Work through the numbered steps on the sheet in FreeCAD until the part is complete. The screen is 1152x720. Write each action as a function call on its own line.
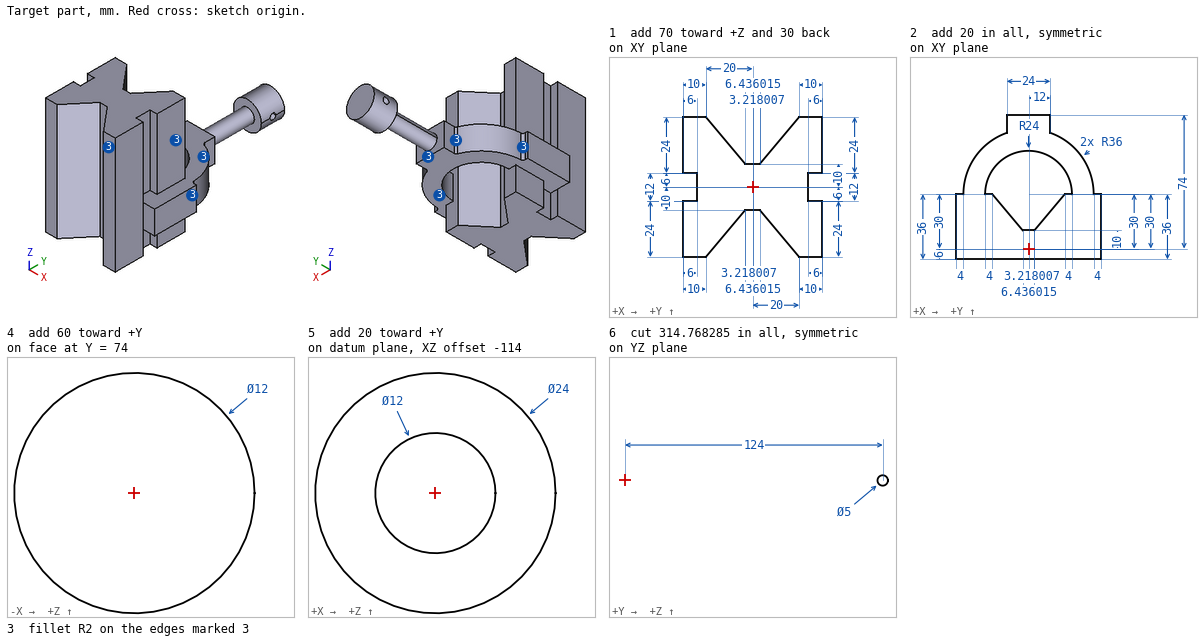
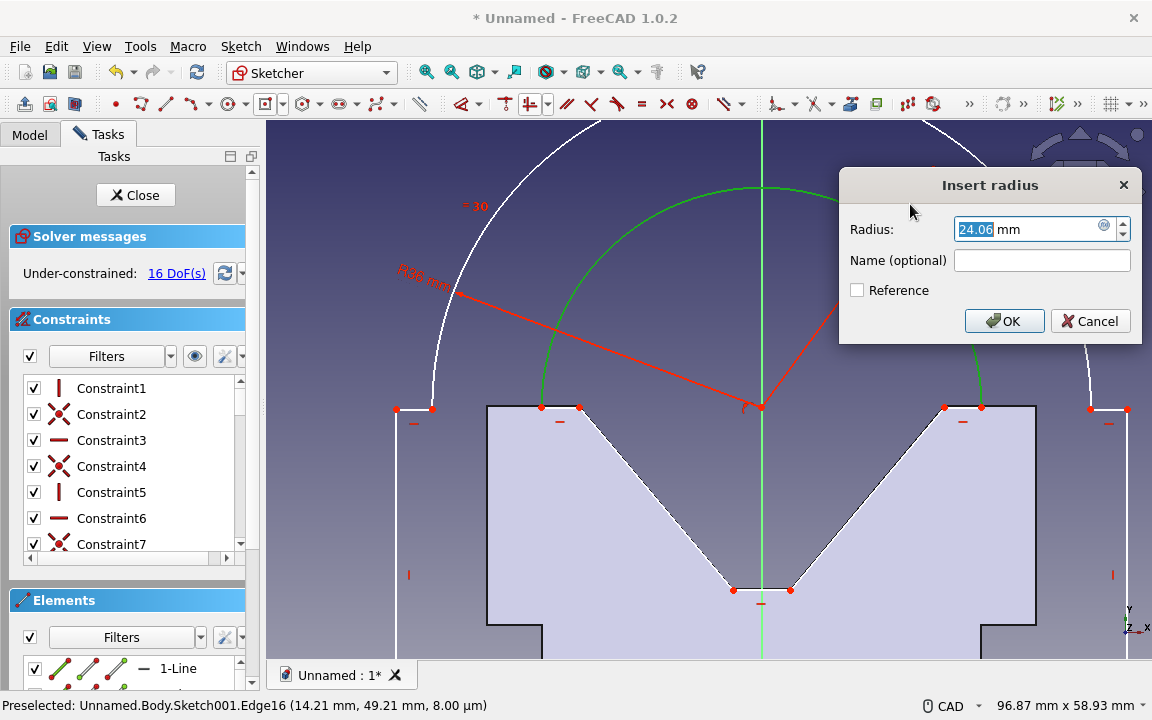
text(24)
key(Return)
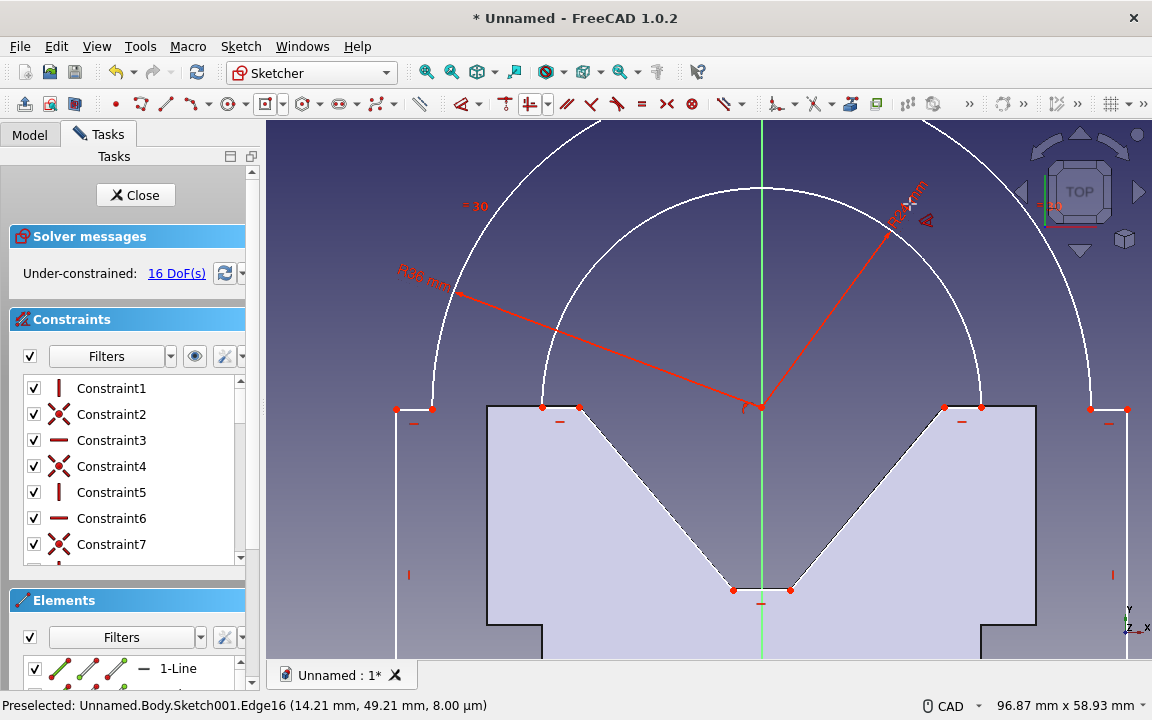
scroll(421, 410, up, 2)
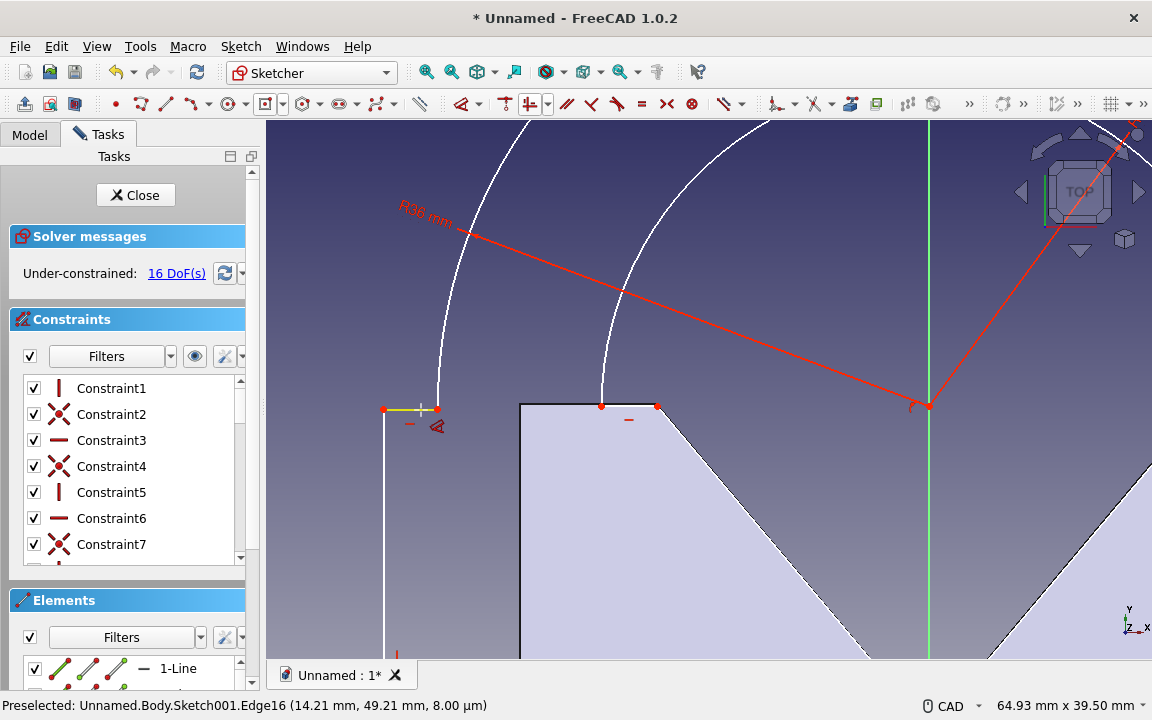
click(422, 410)
click(411, 444)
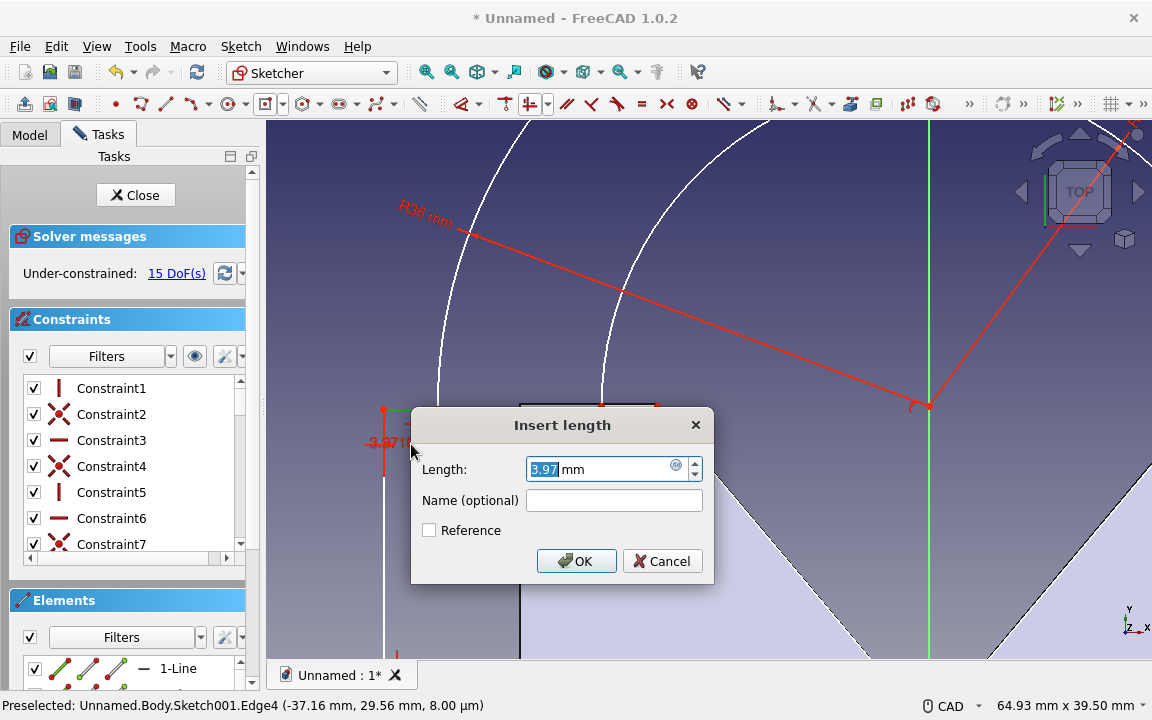
text(4)
key(Return)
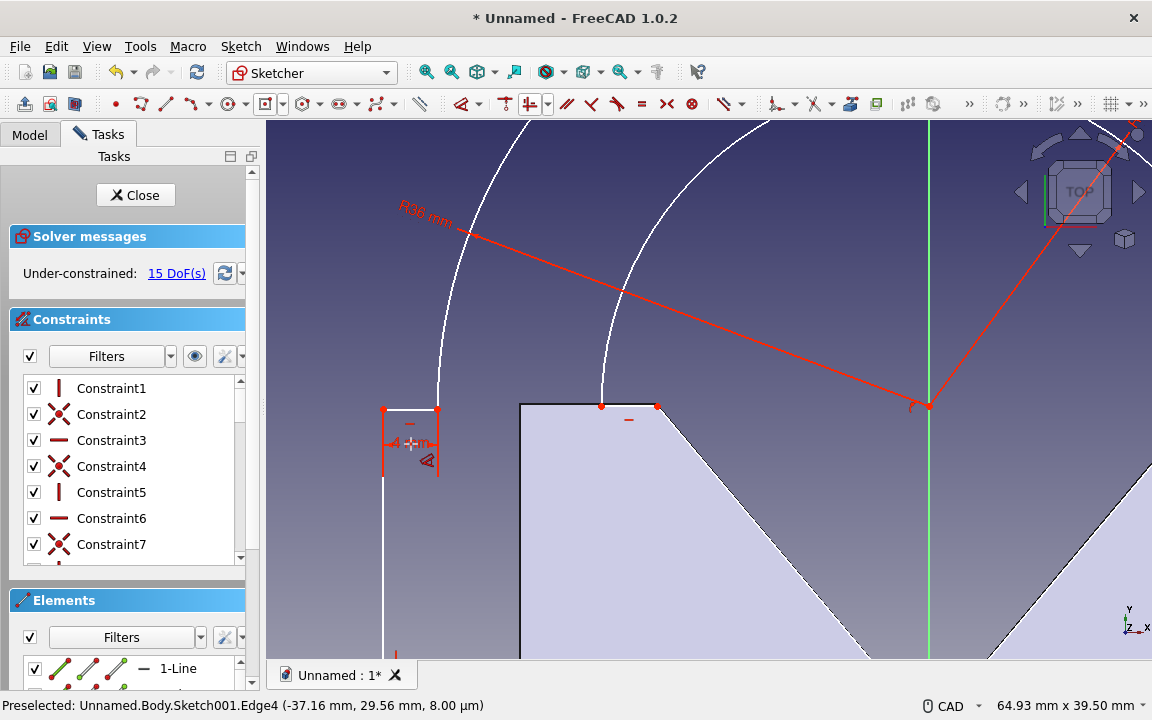
scroll(516, 407, down, 6)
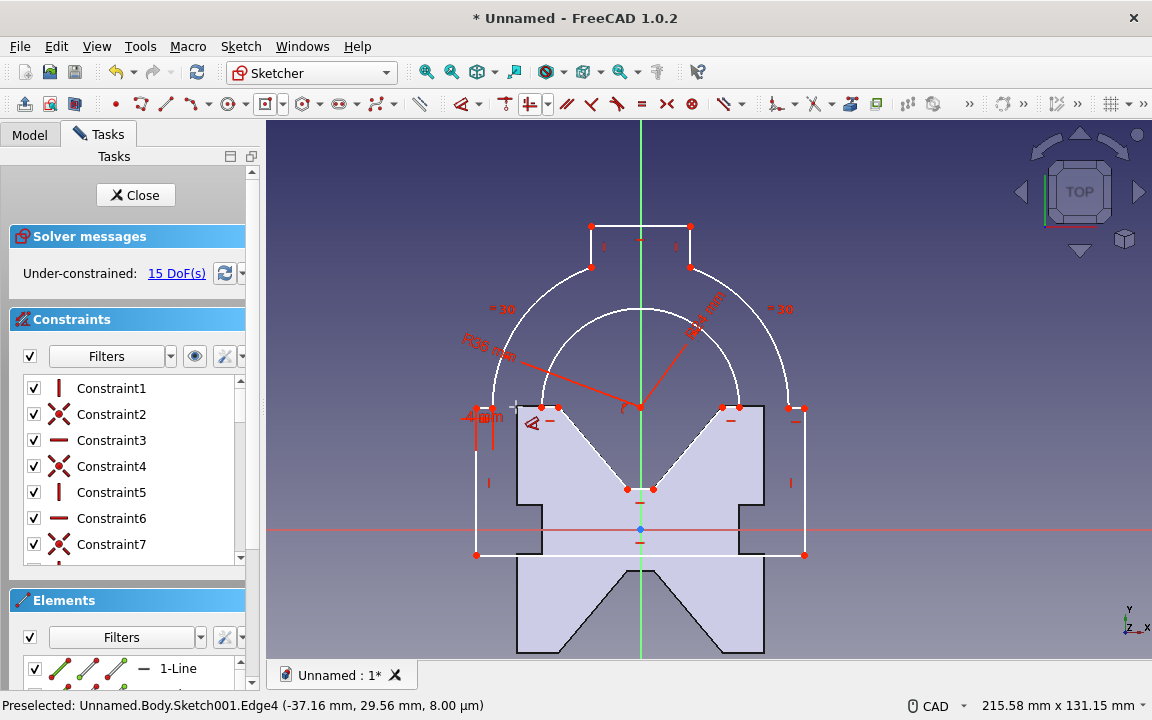
scroll(800, 408, up, 6)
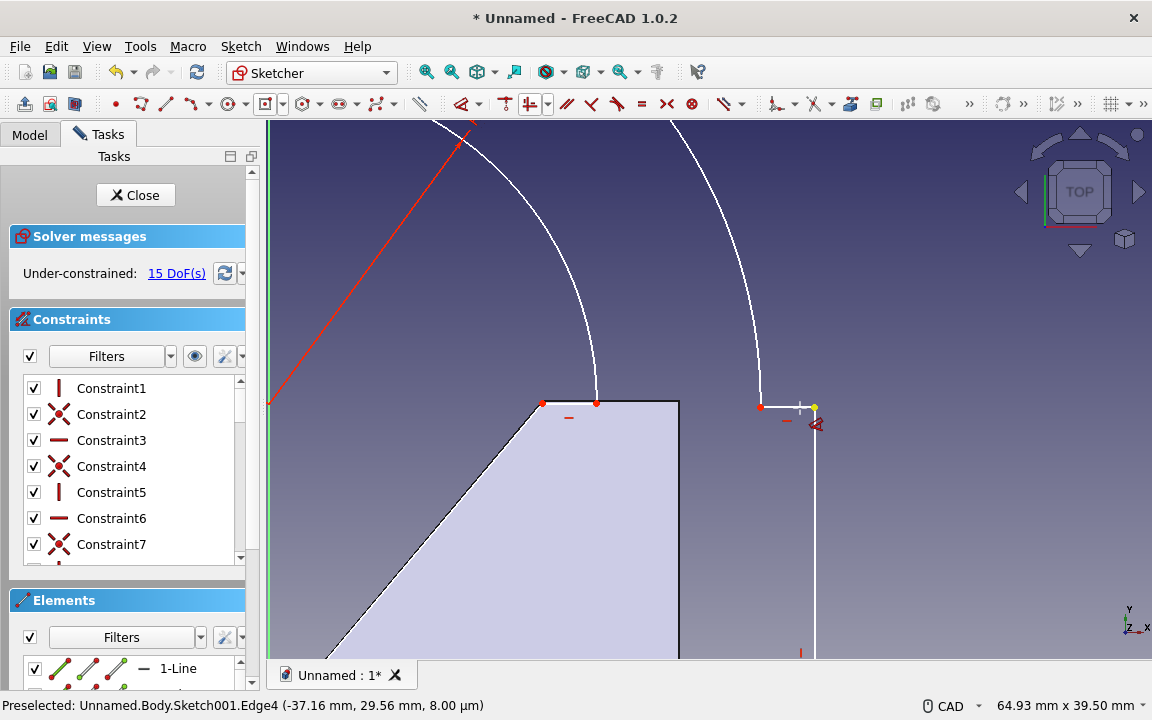
click(799, 407)
click(788, 441)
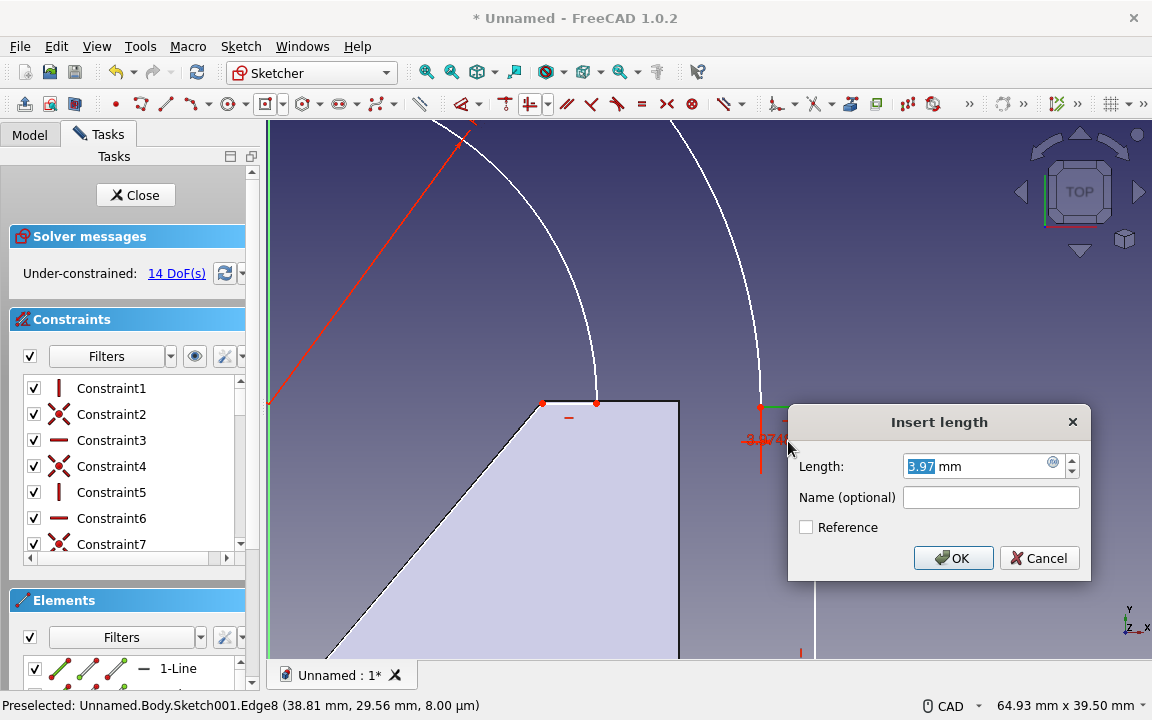
text(4)
key(Return)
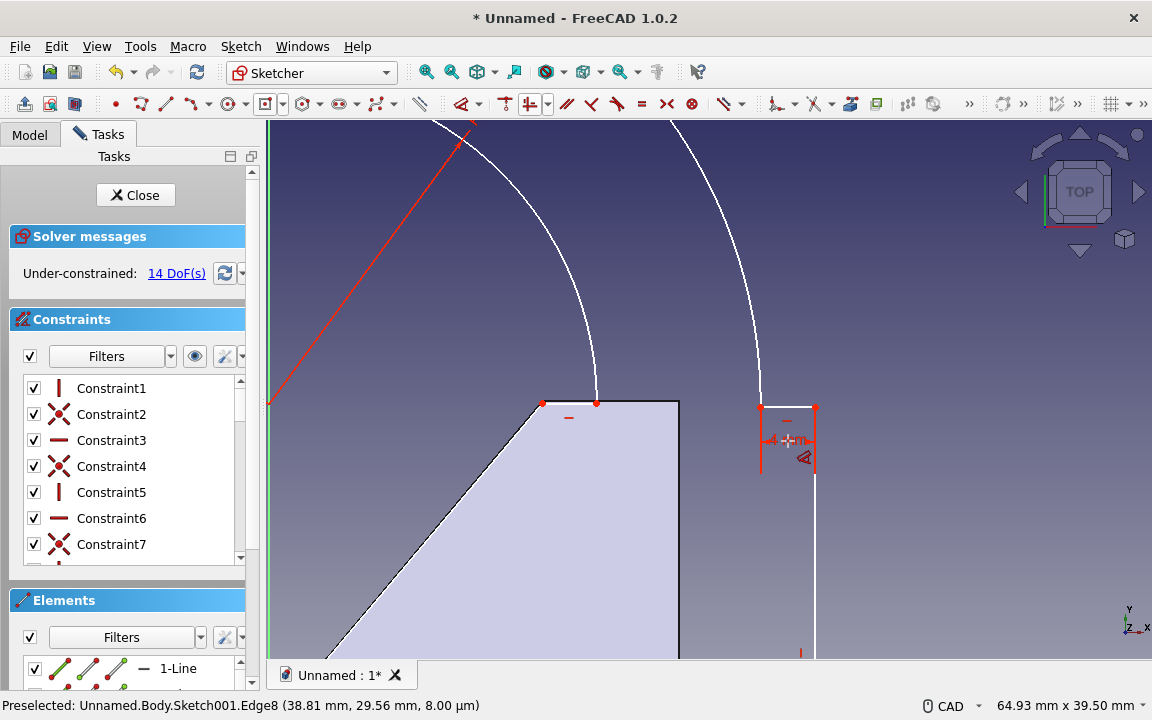
click(580, 404)
click(570, 438)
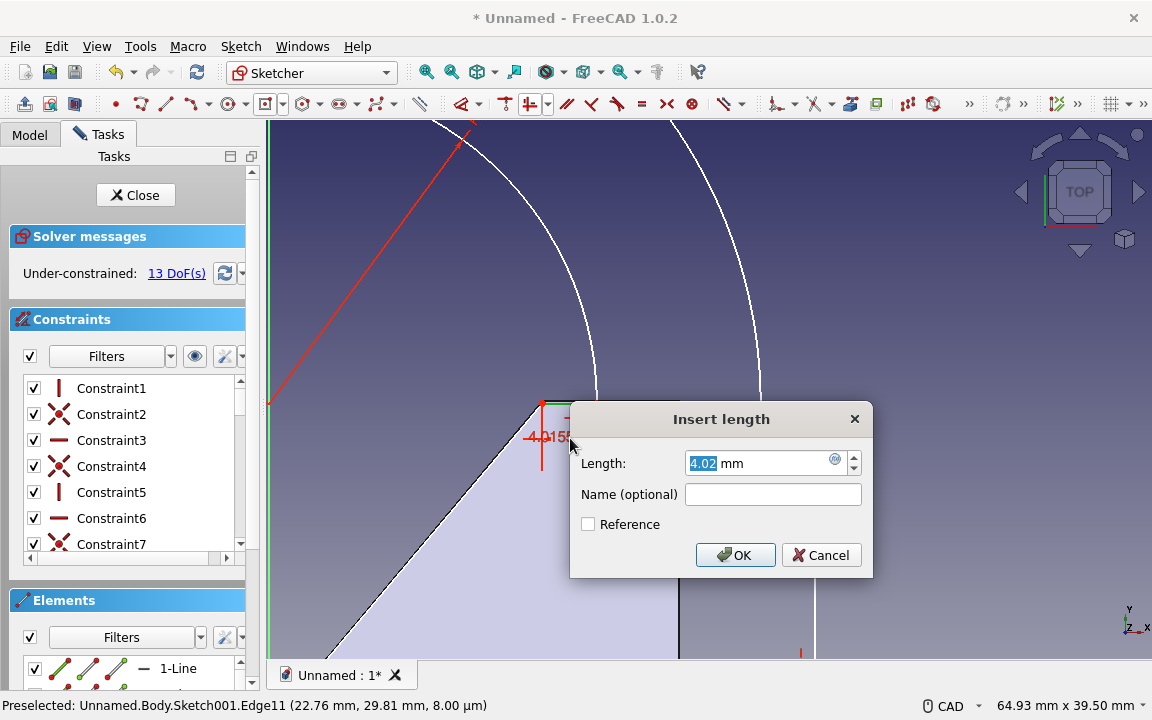
text(4)
key(Return)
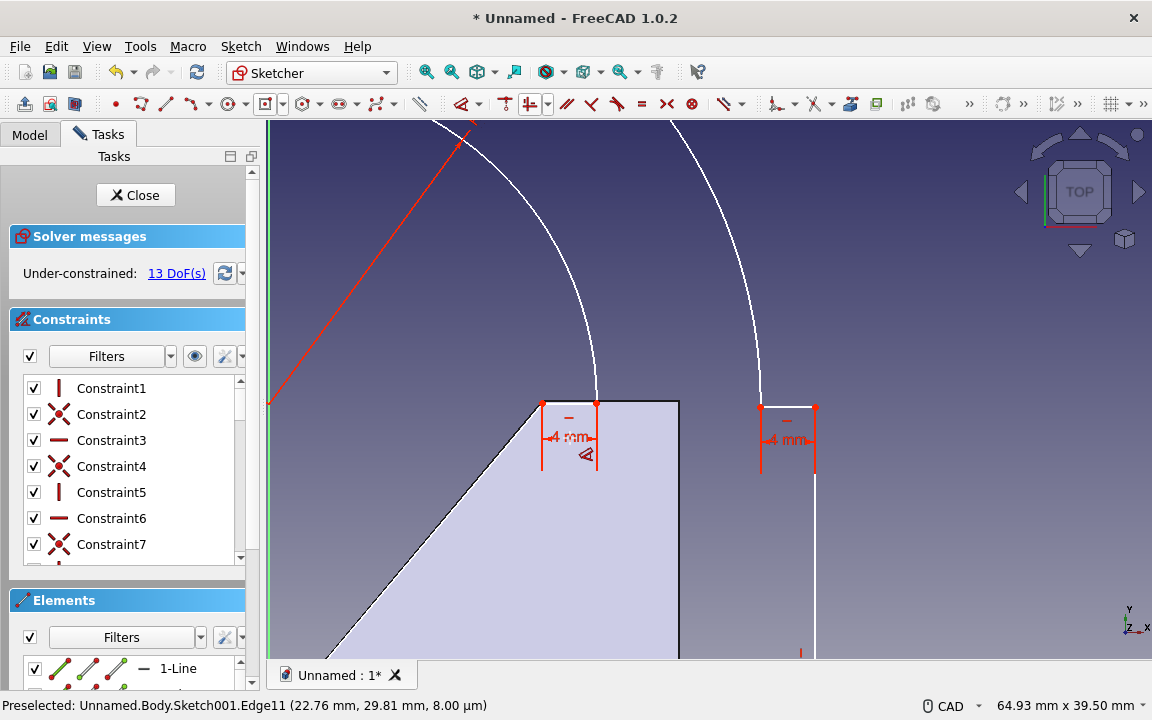
scroll(800, 408, down, 6)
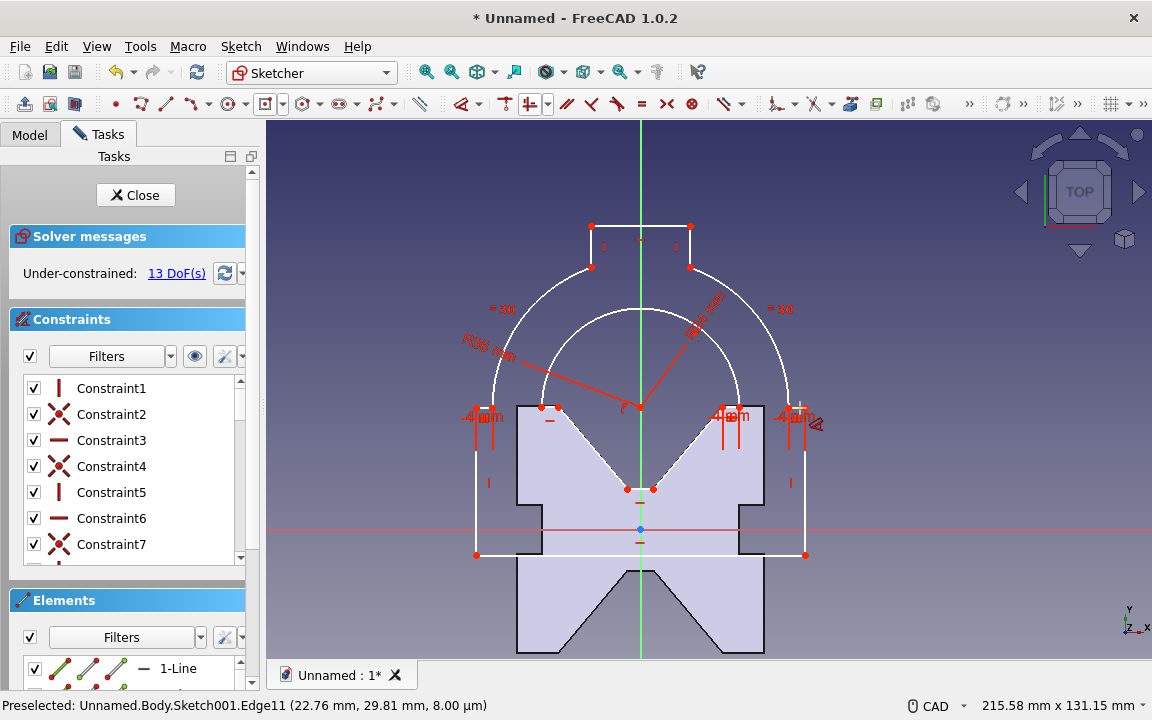
scroll(554, 407, up, 6)